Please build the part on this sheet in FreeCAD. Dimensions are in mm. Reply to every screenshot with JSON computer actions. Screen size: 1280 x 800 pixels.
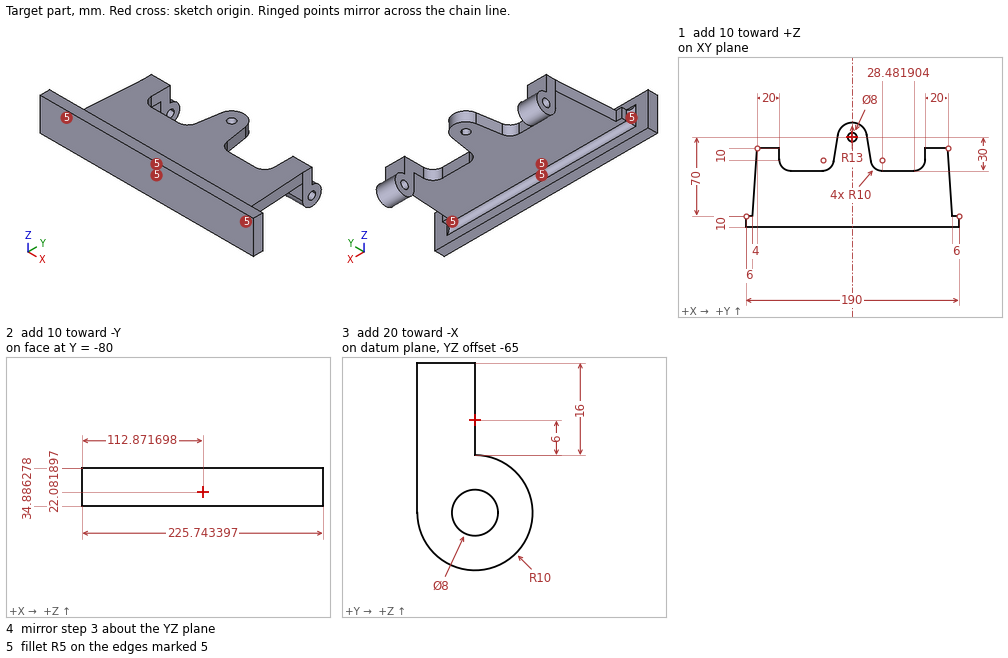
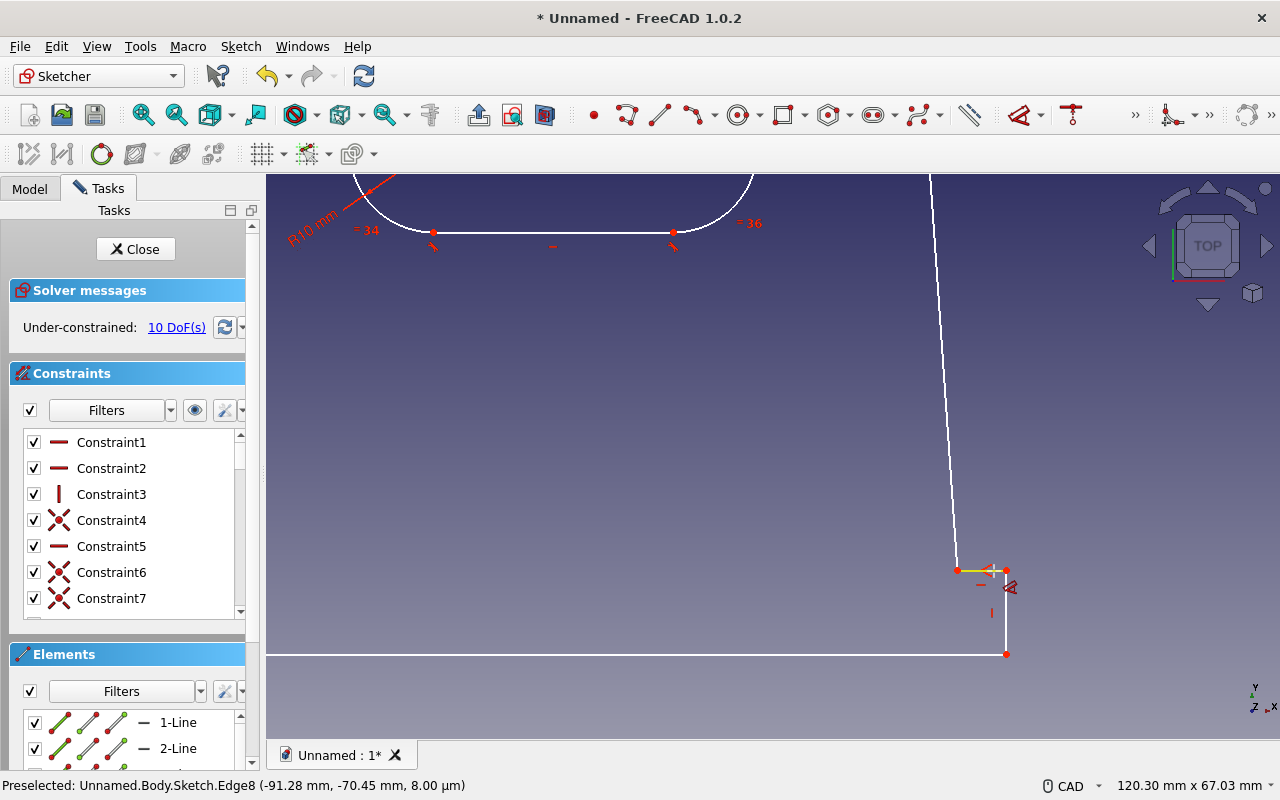
{"action": "left_click", "coordinate": [992, 571]}
{"action": "left_click", "coordinate": [982, 605]}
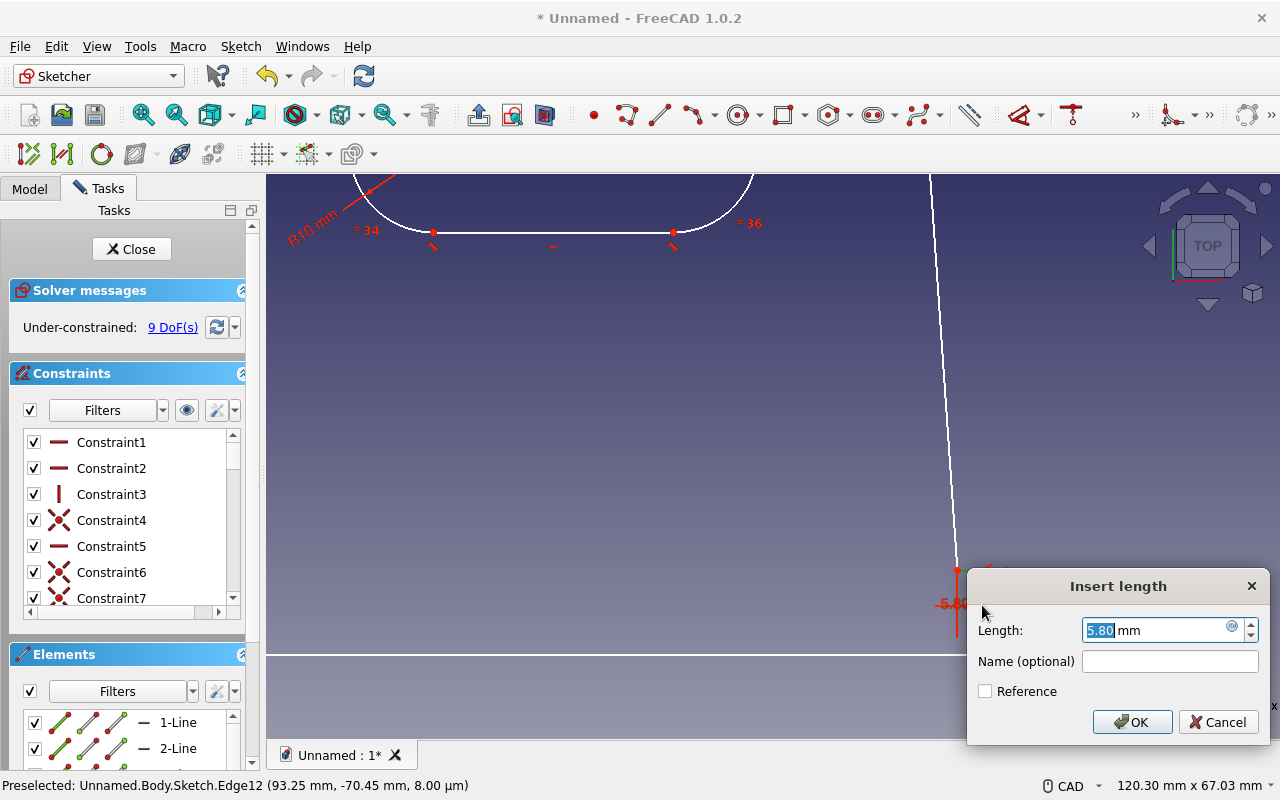
{"action": "type", "text": "6"}
{"action": "key", "text": "Return"}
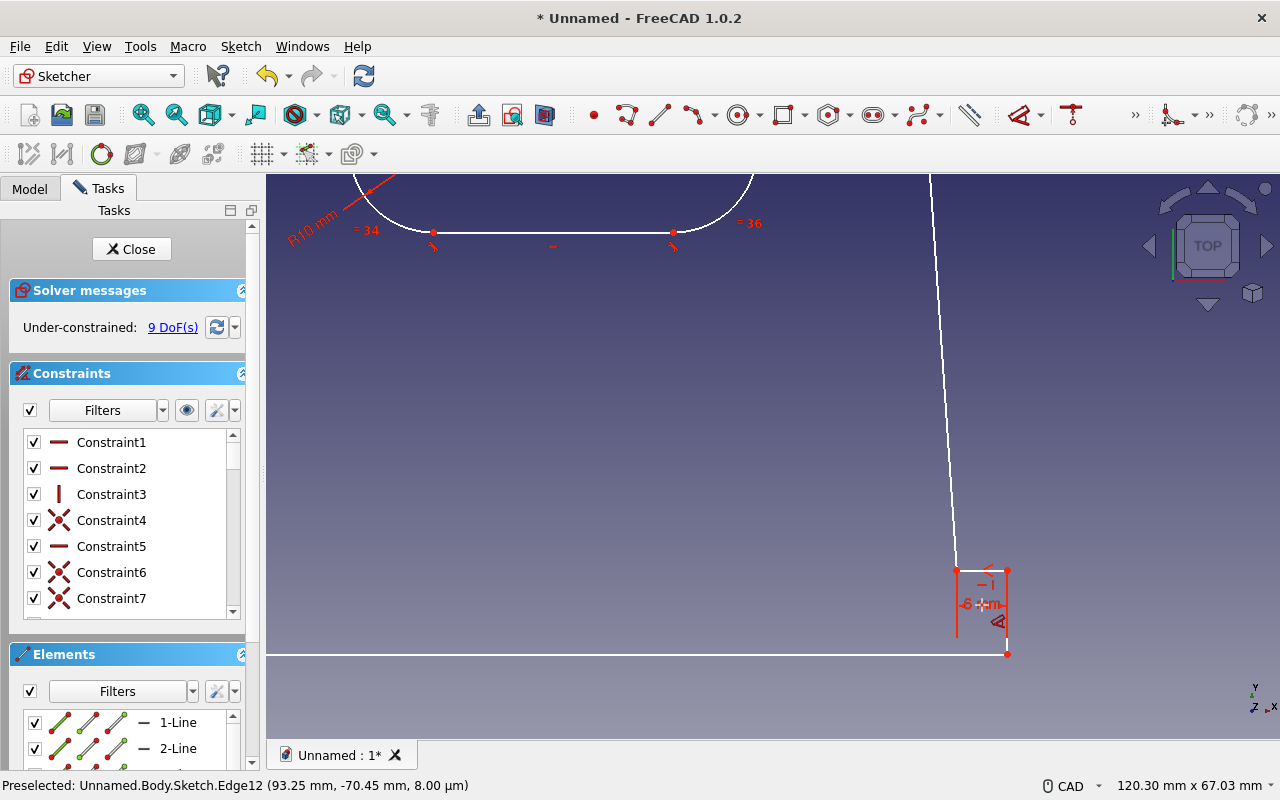
{"action": "scroll", "coordinate": [995, 571], "scroll_direction": "down", "scroll_amount": 5}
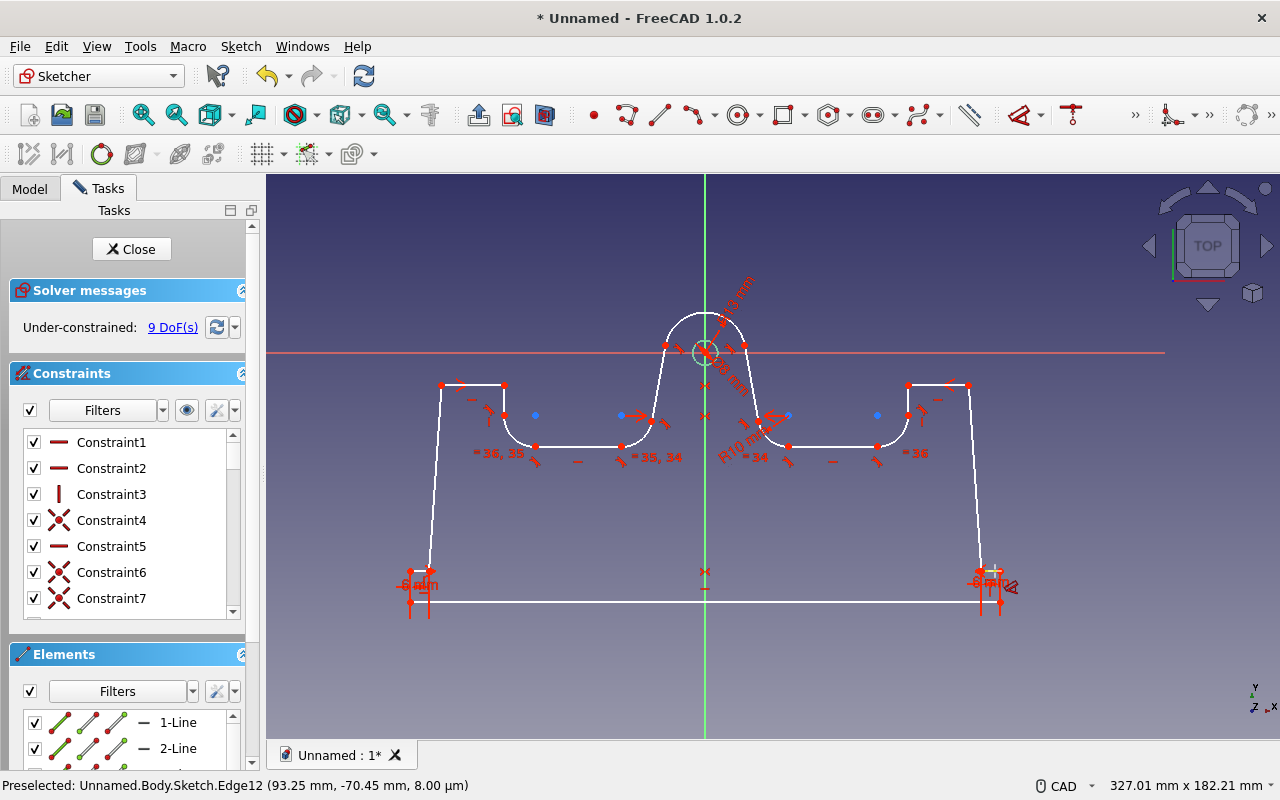
{"action": "scroll", "coordinate": [504, 407], "scroll_direction": "up", "scroll_amount": 3}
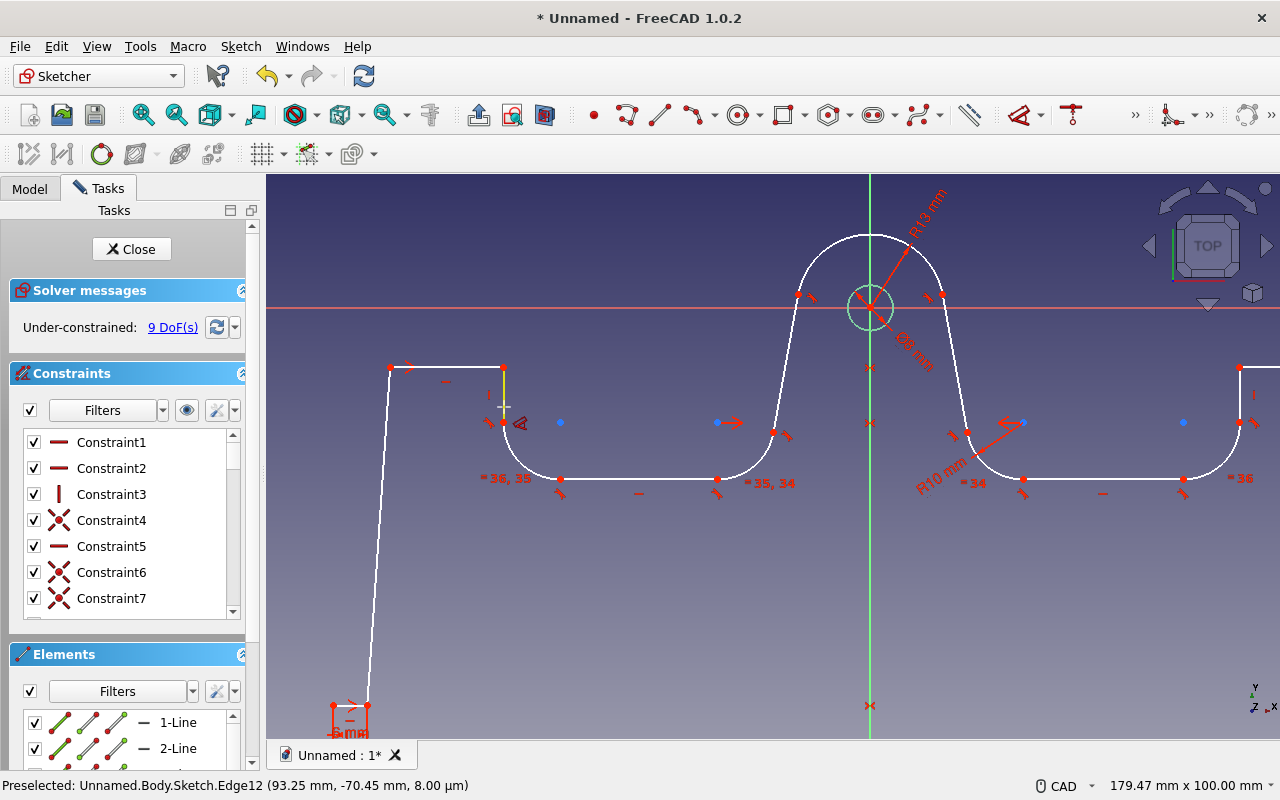
{"action": "left_click", "coordinate": [504, 406]}
{"action": "left_click", "coordinate": [470, 395]}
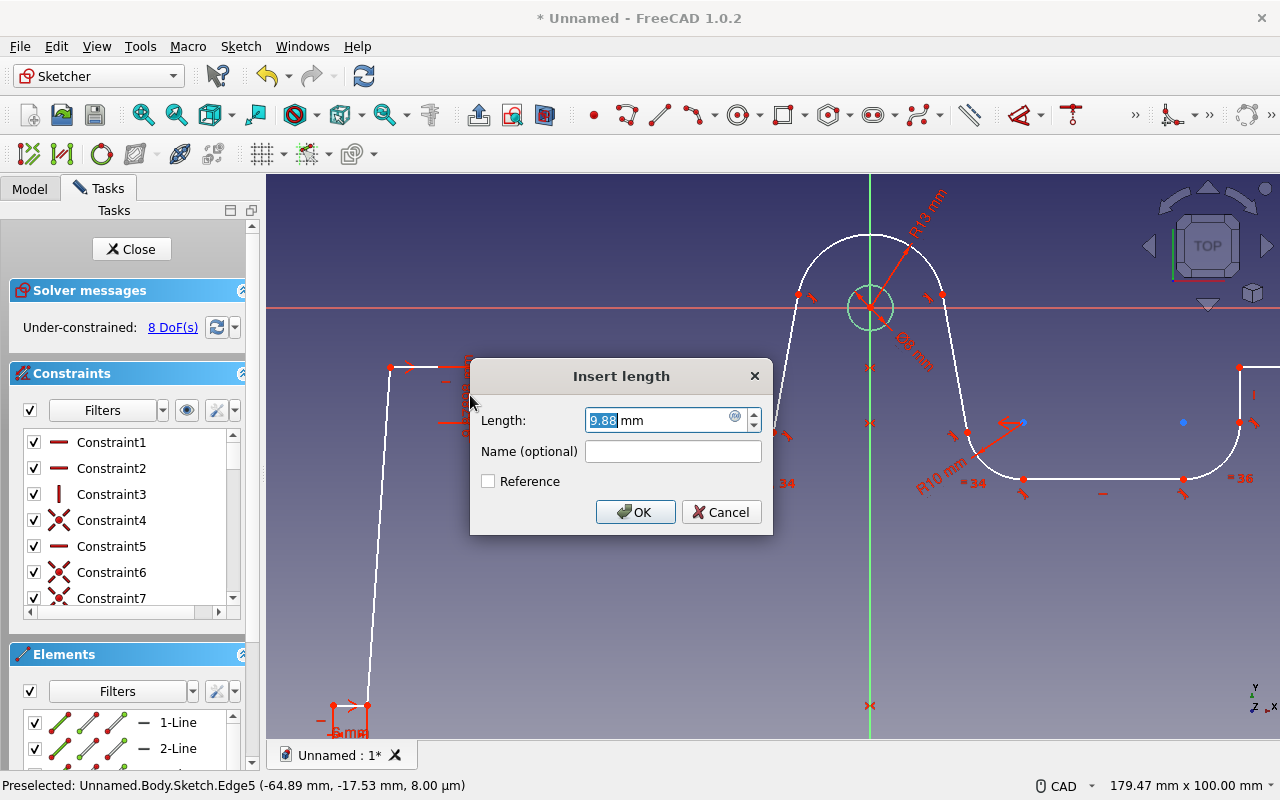
{"action": "type", "text": "10"}
{"action": "key", "text": "Return"}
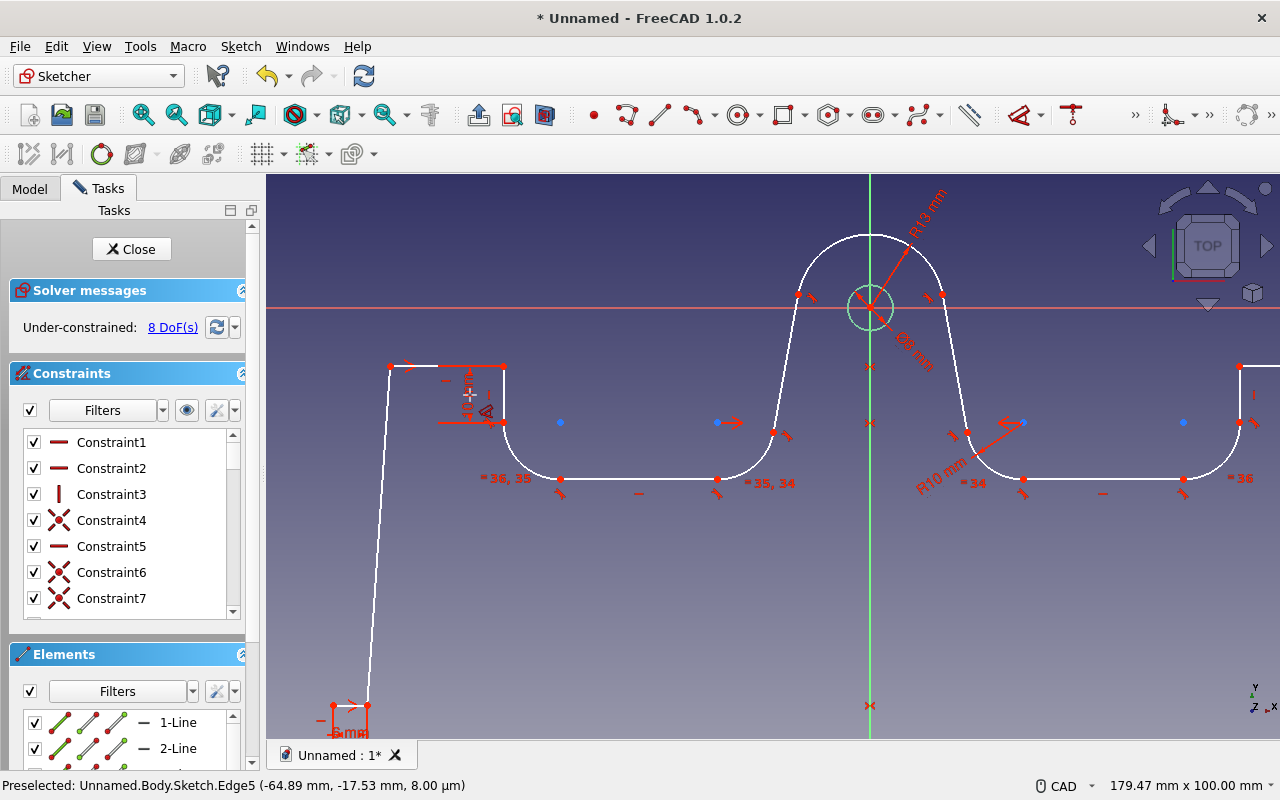
{"action": "left_click", "coordinate": [470, 366]}
{"action": "left_click", "coordinate": [447, 332]}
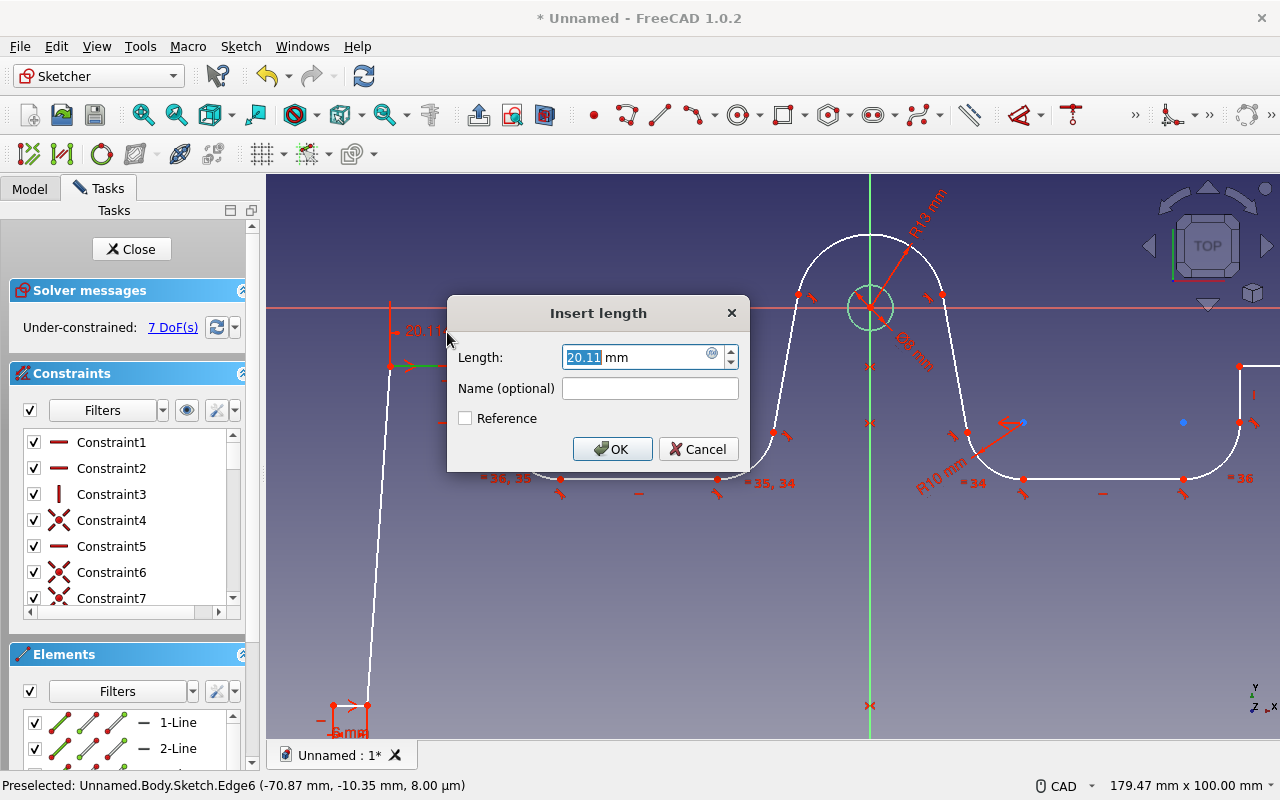
{"action": "type", "text": "20"}
{"action": "key", "text": "Return"}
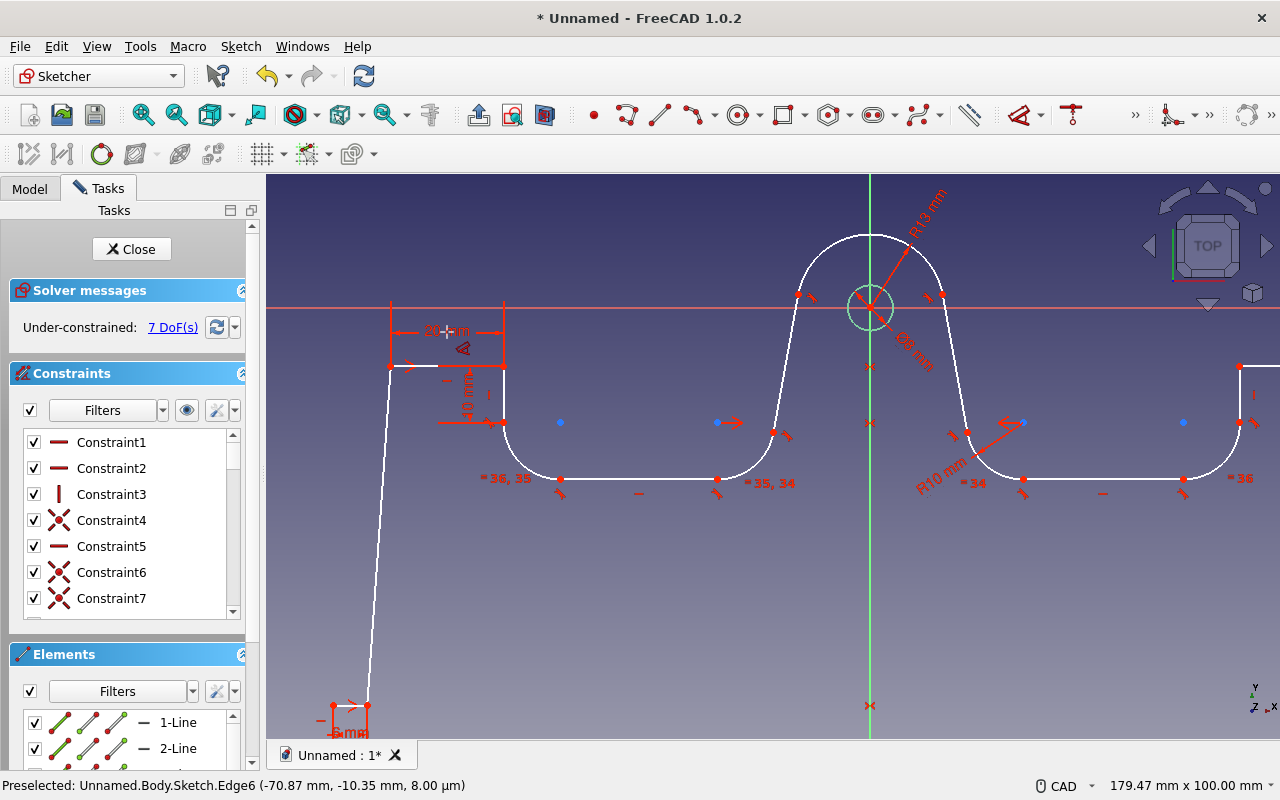
{"action": "scroll", "coordinate": [503, 407], "scroll_direction": "down", "scroll_amount": 3}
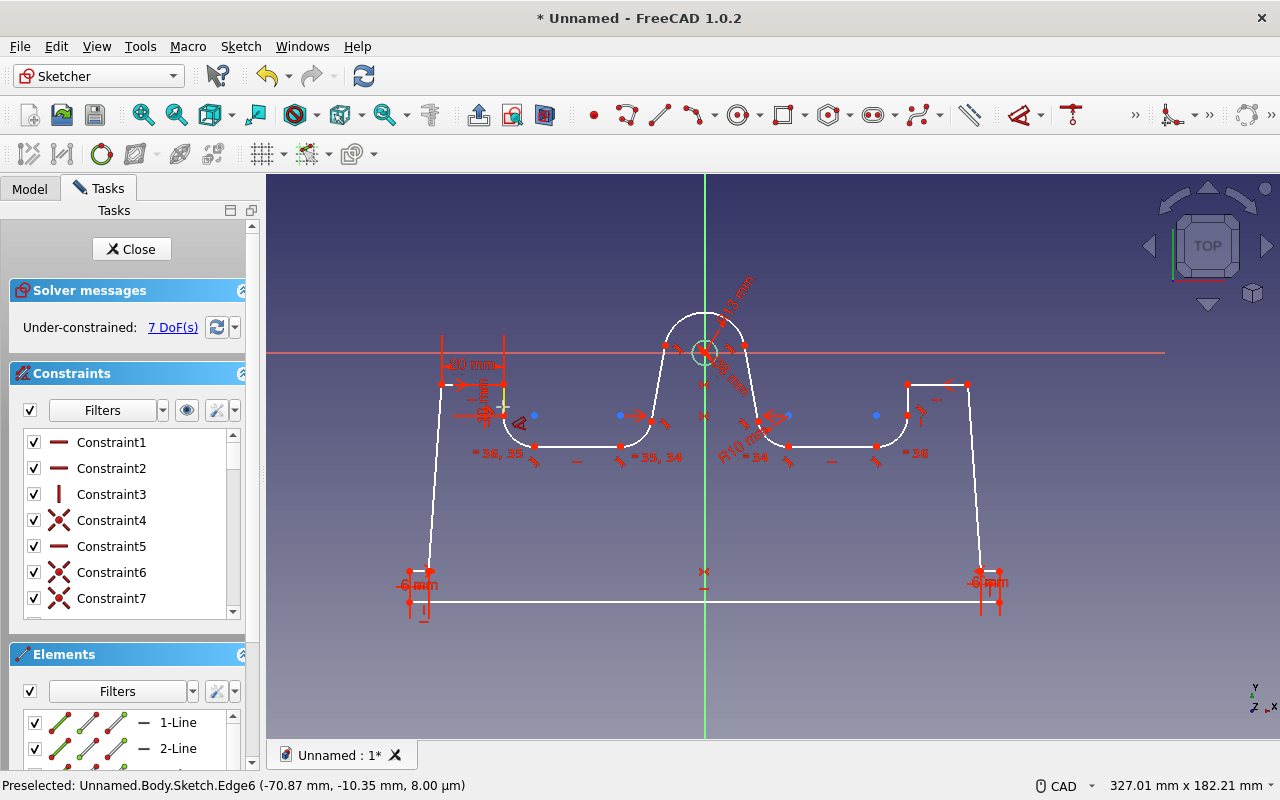
{"action": "scroll", "coordinate": [410, 581], "scroll_direction": "up", "scroll_amount": 2}